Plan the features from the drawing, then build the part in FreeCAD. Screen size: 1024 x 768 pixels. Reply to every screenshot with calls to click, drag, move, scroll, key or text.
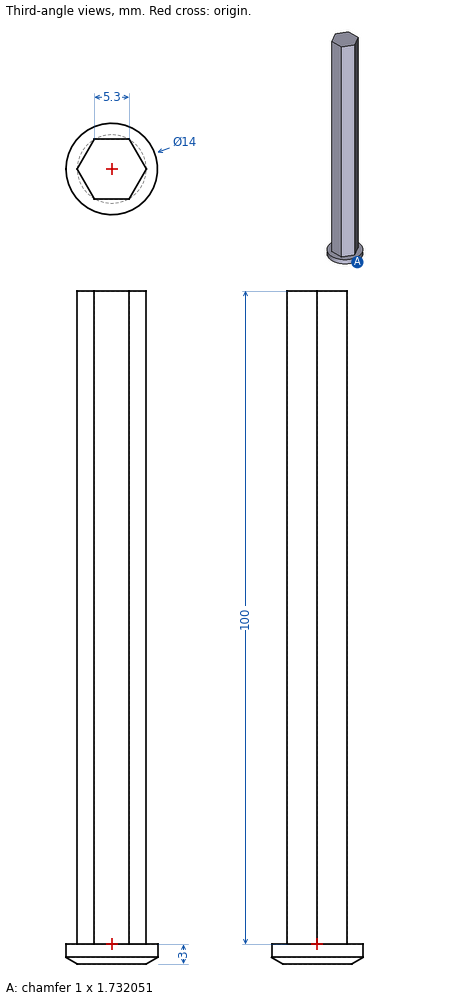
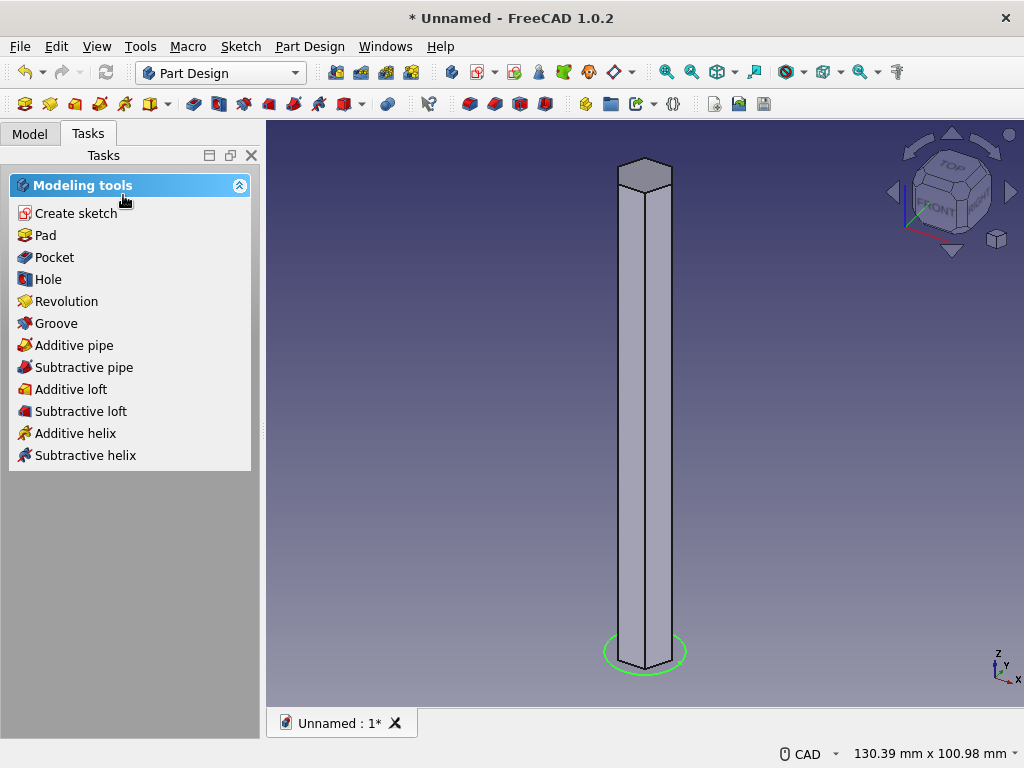
click(25, 104)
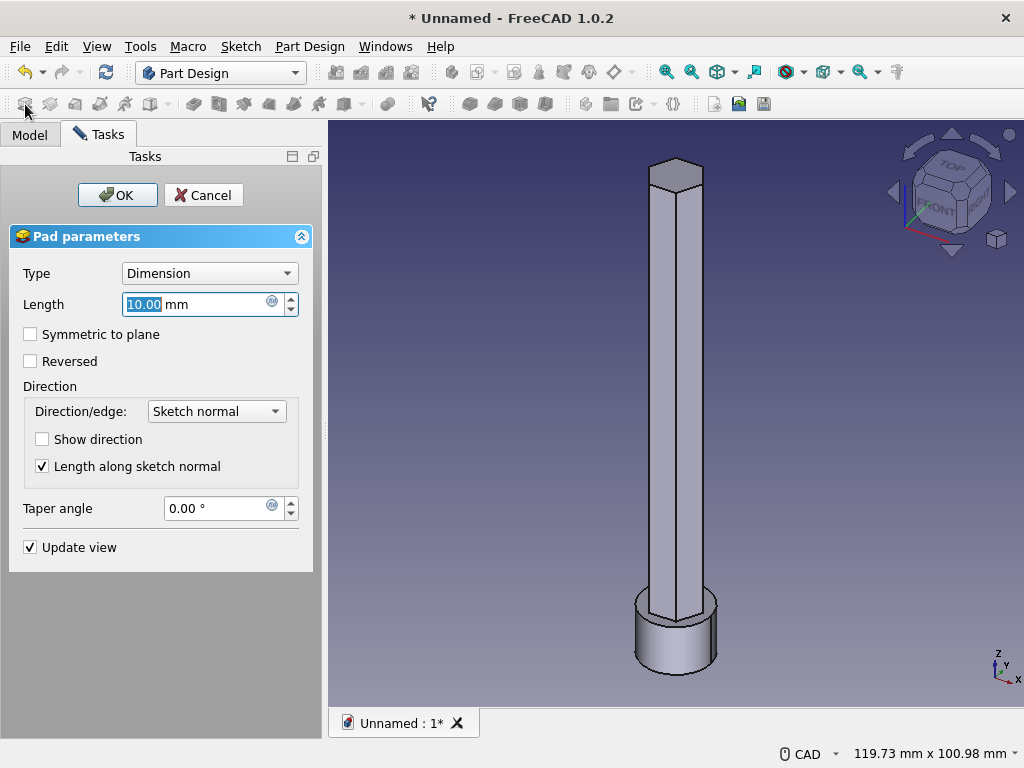
text(3)
key(Tab)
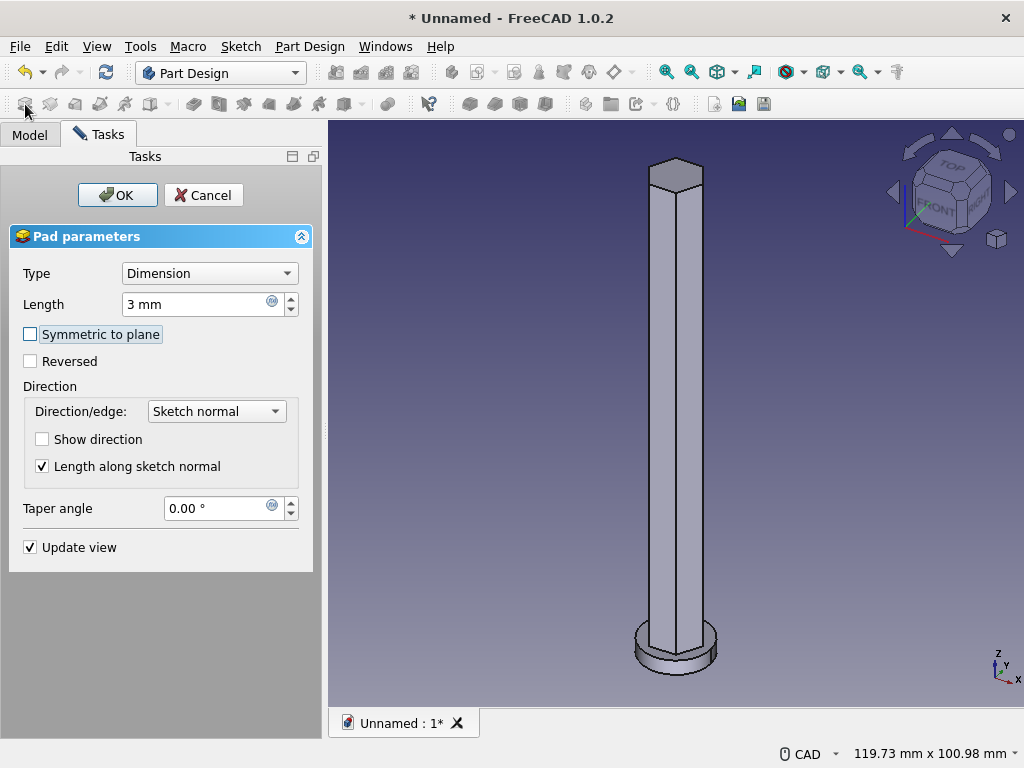
click(31, 361)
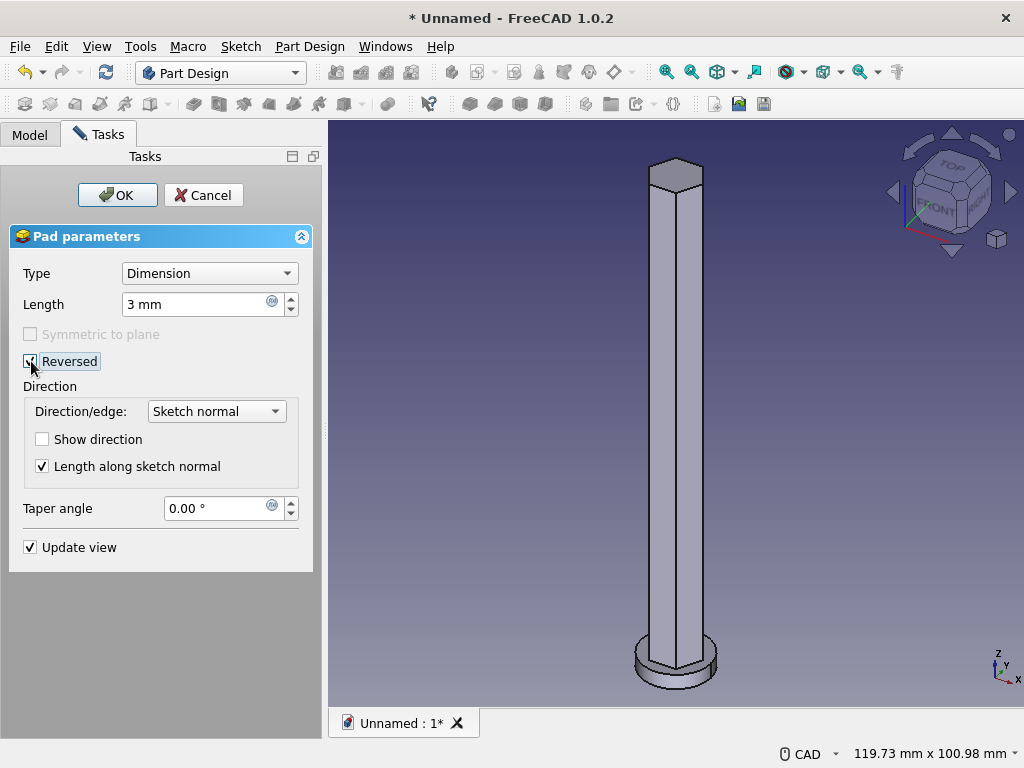
click(118, 195)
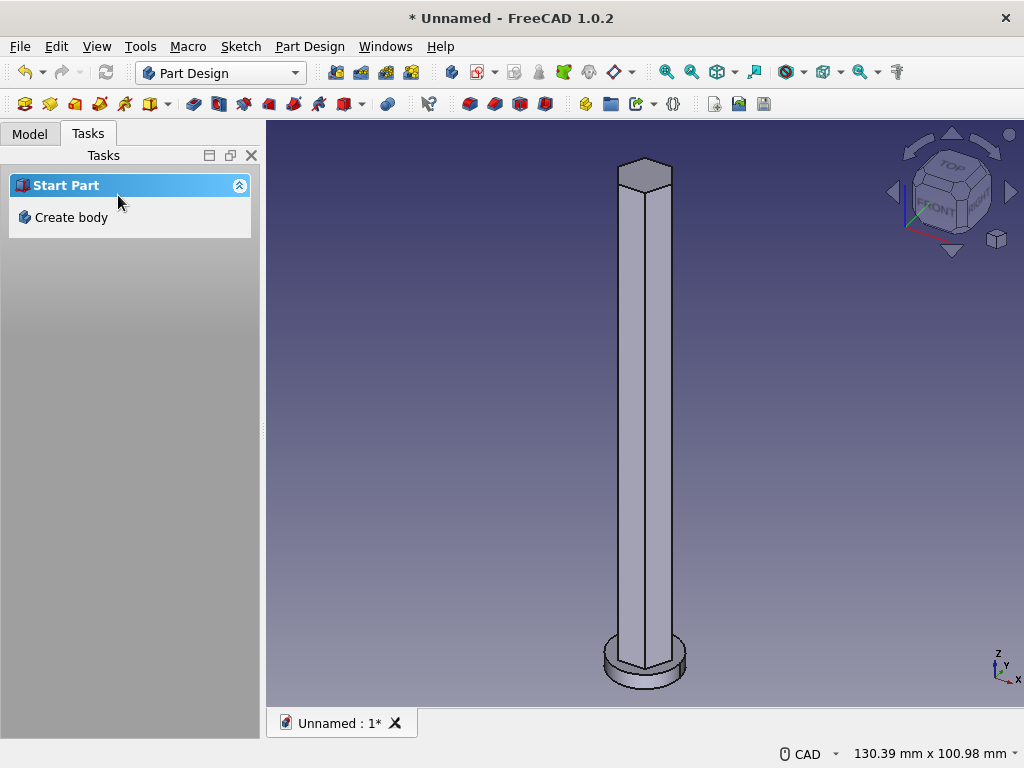
key(0)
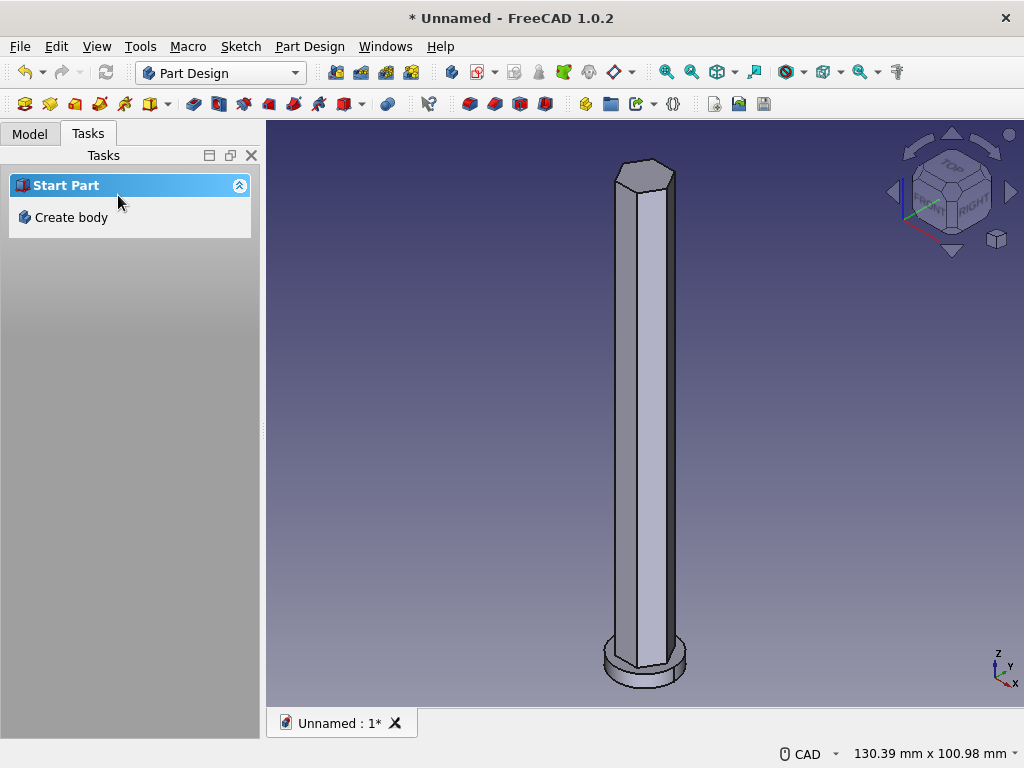
key(2)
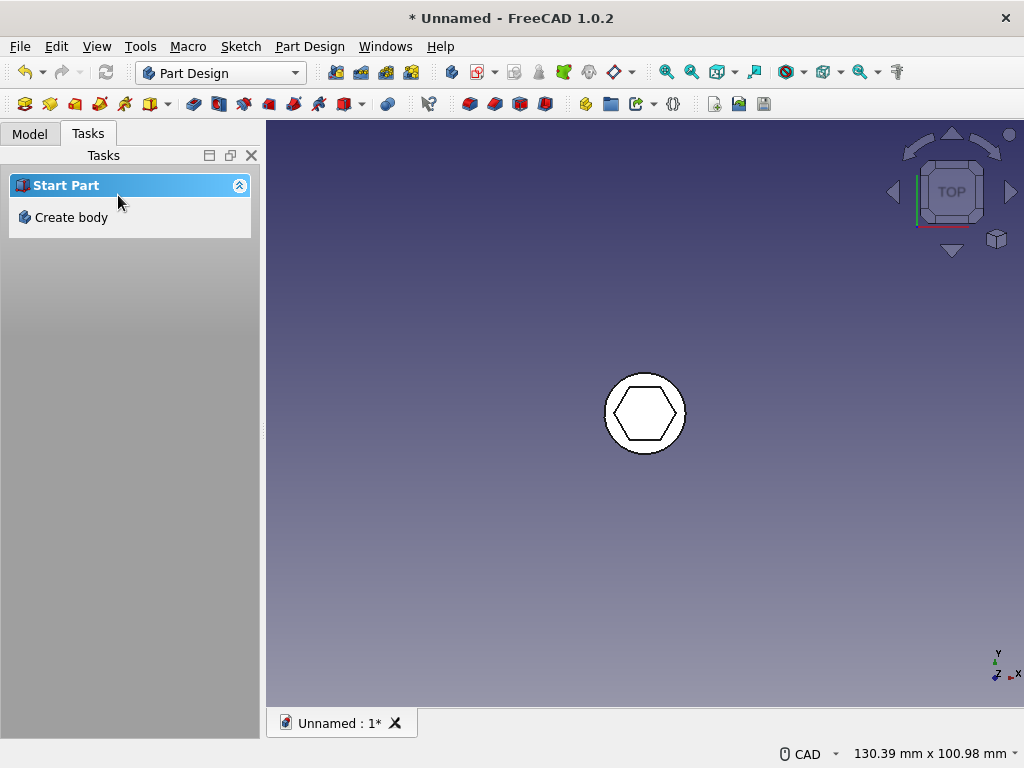
click(667, 72)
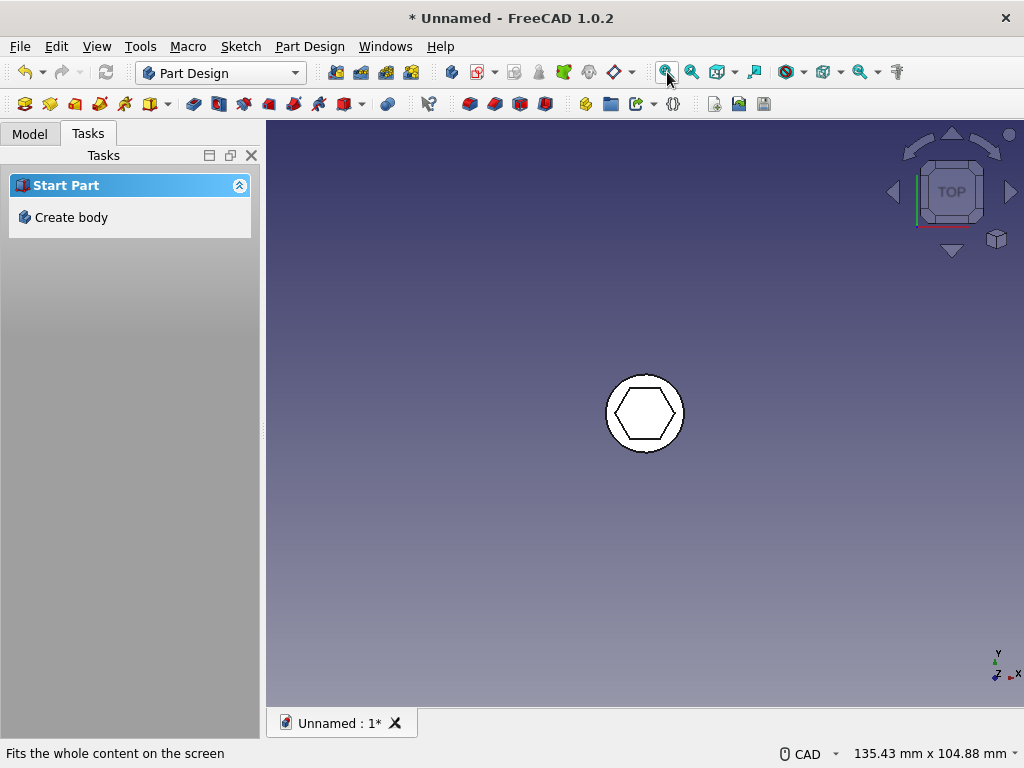
key(1)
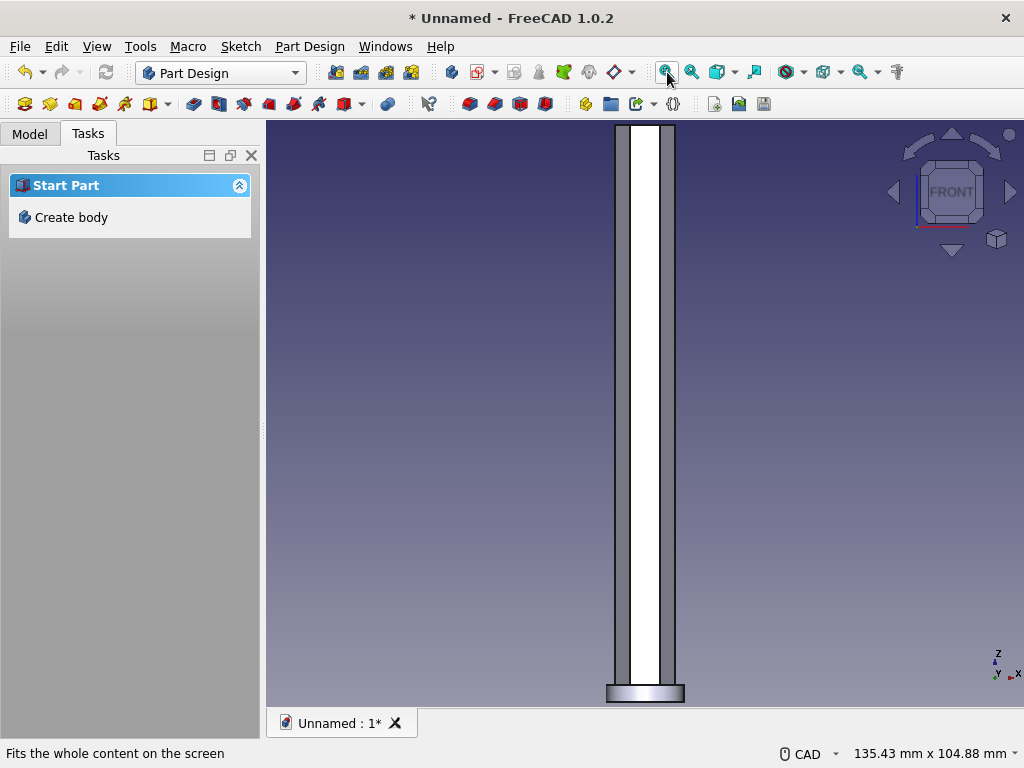
key(3)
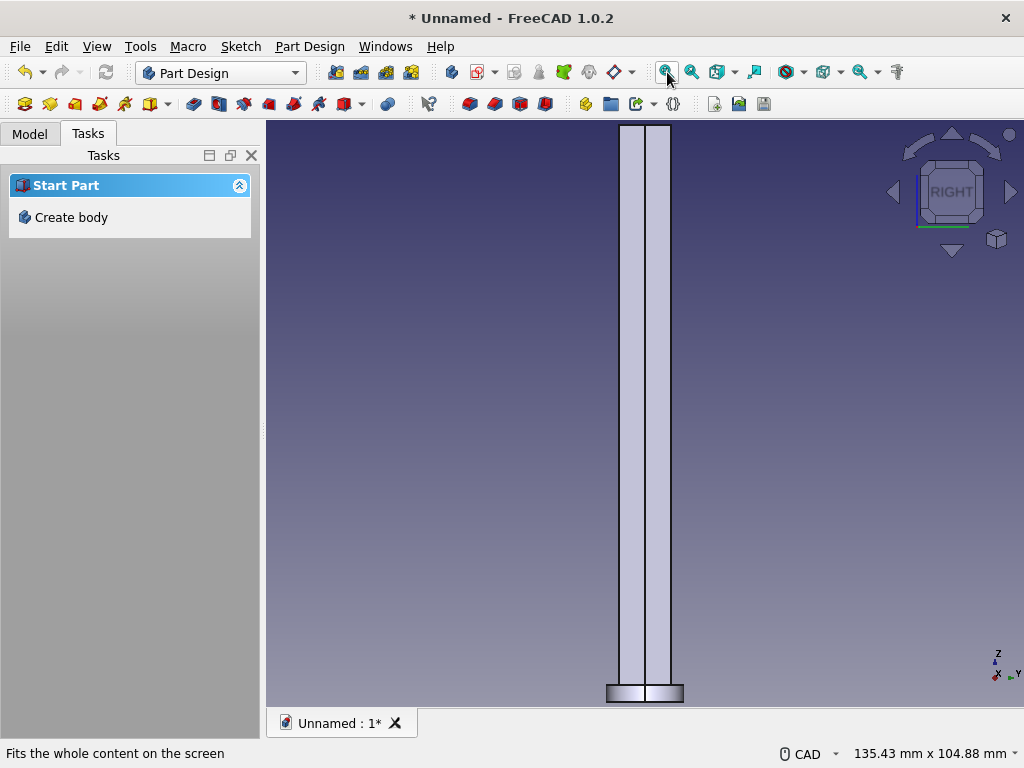
key(5)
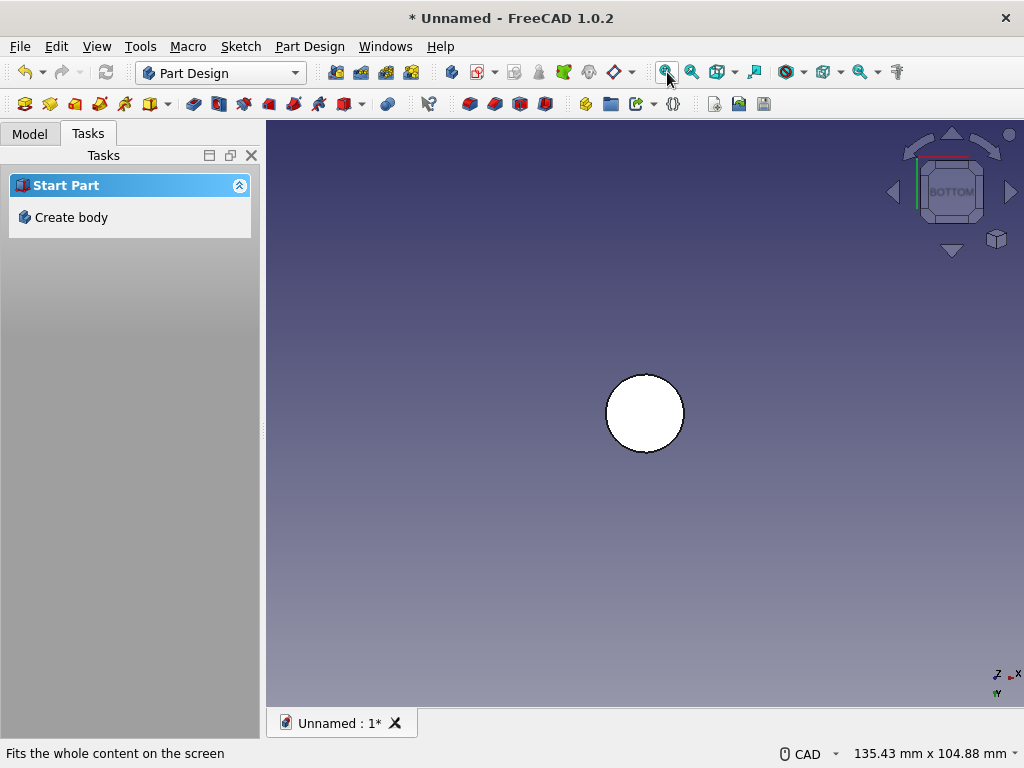
click(667, 72)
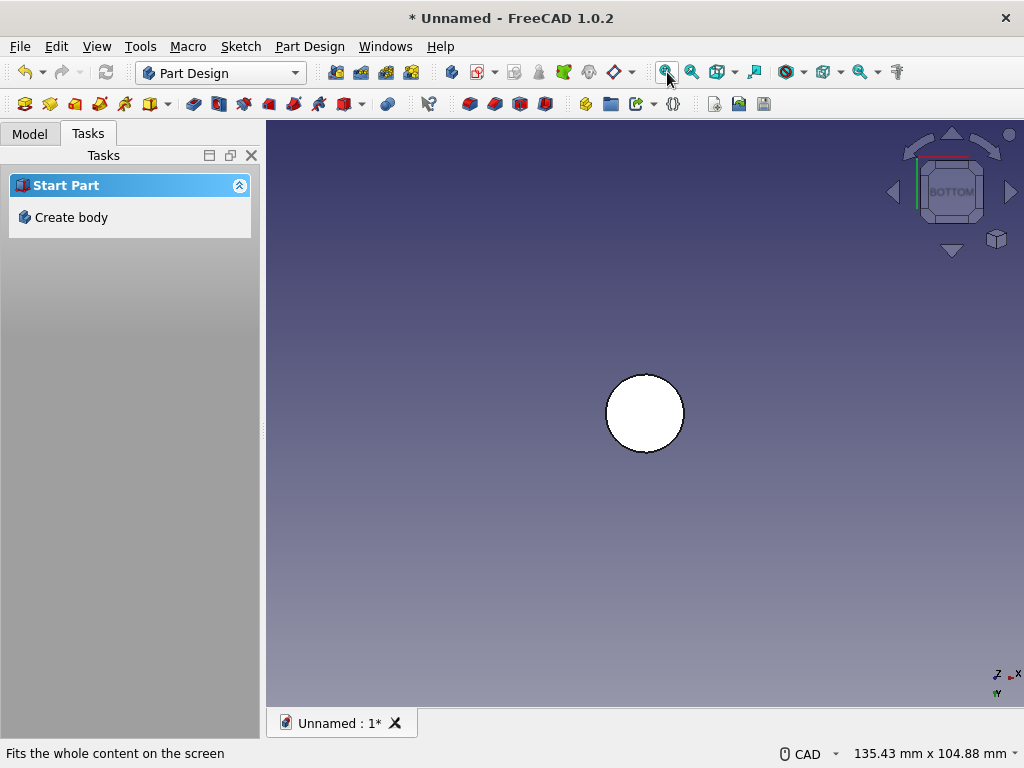
click(606, 412)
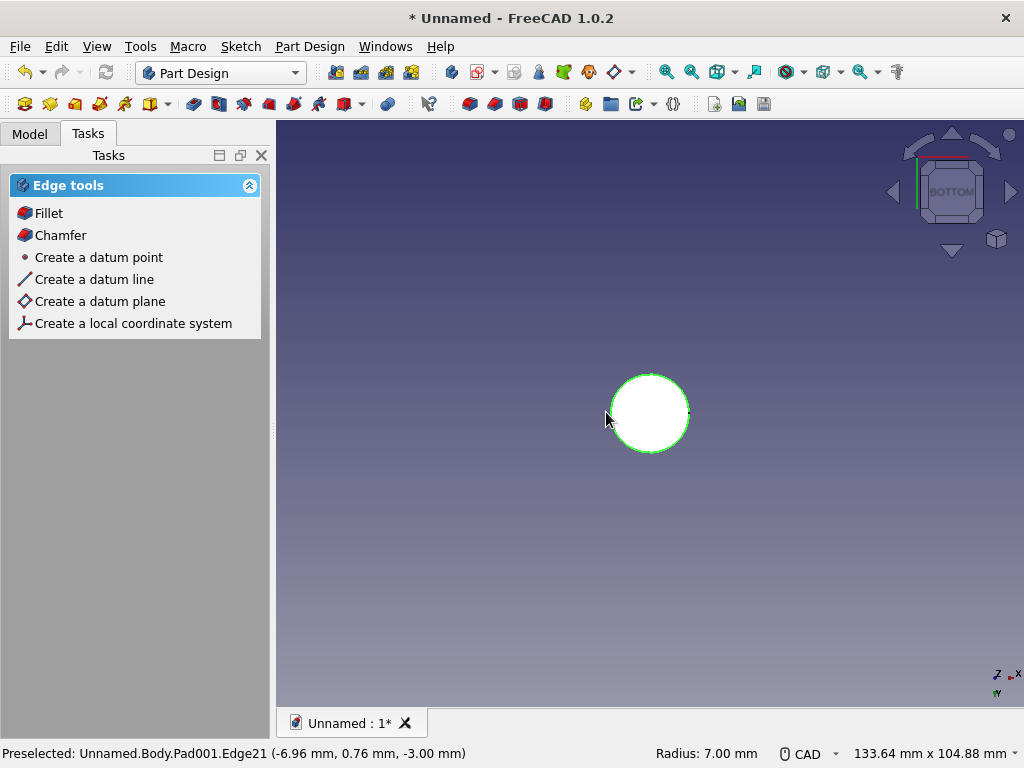
click(495, 104)